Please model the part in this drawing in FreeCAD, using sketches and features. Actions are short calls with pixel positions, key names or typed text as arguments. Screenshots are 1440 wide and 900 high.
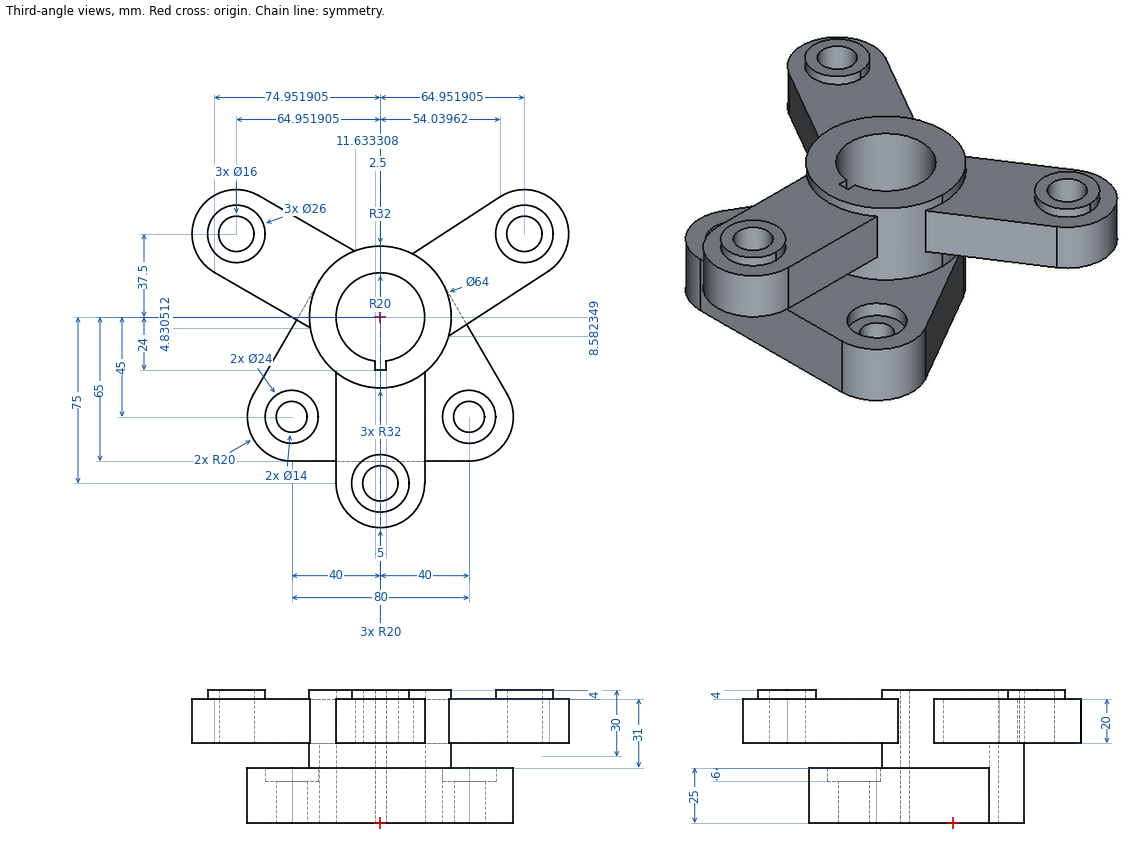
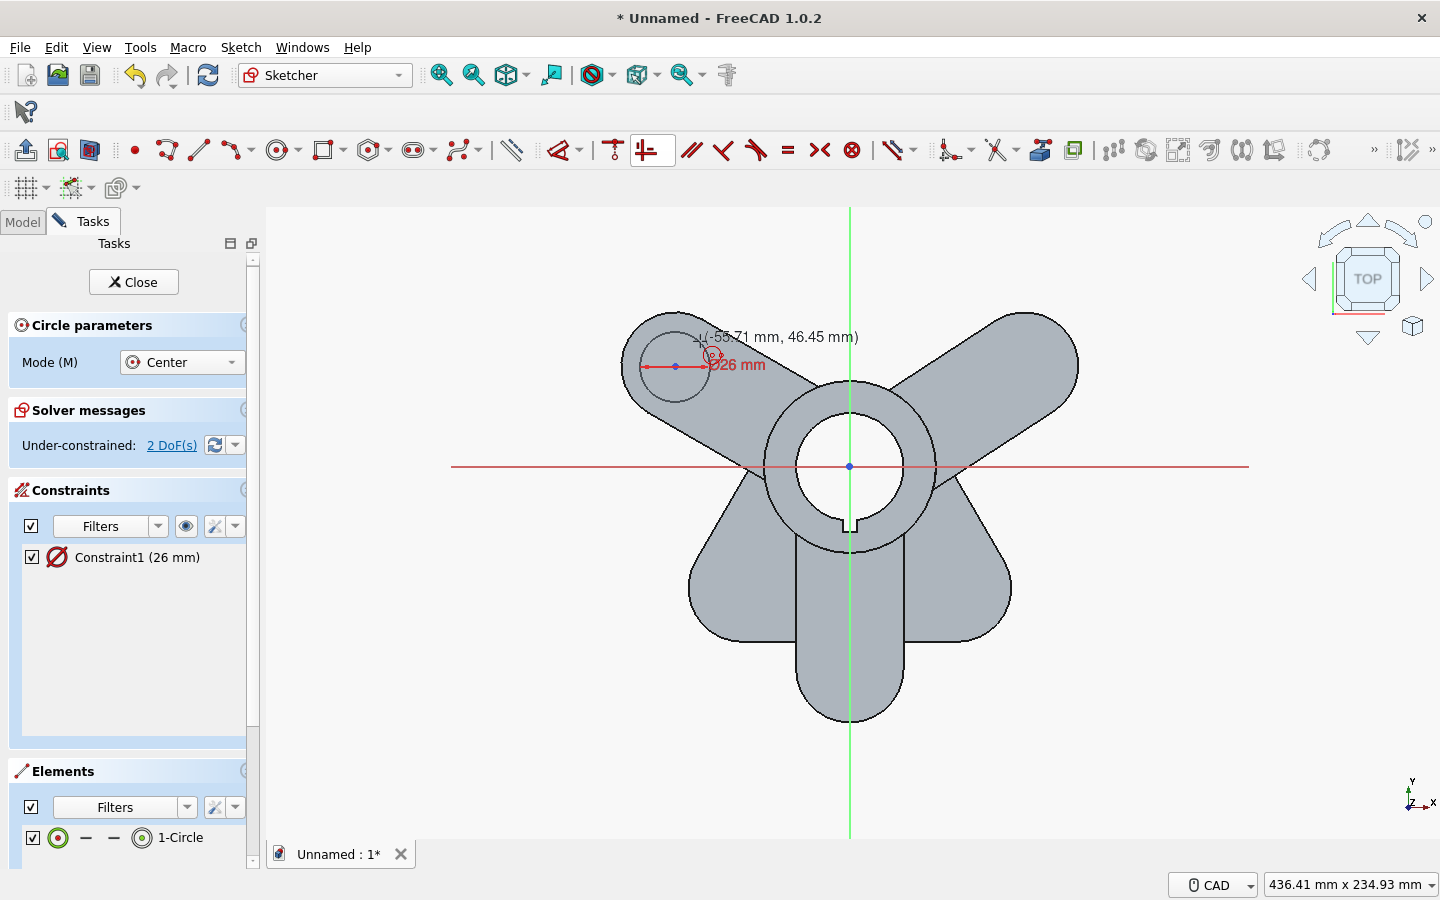
click(1025, 366)
move(1049, 341)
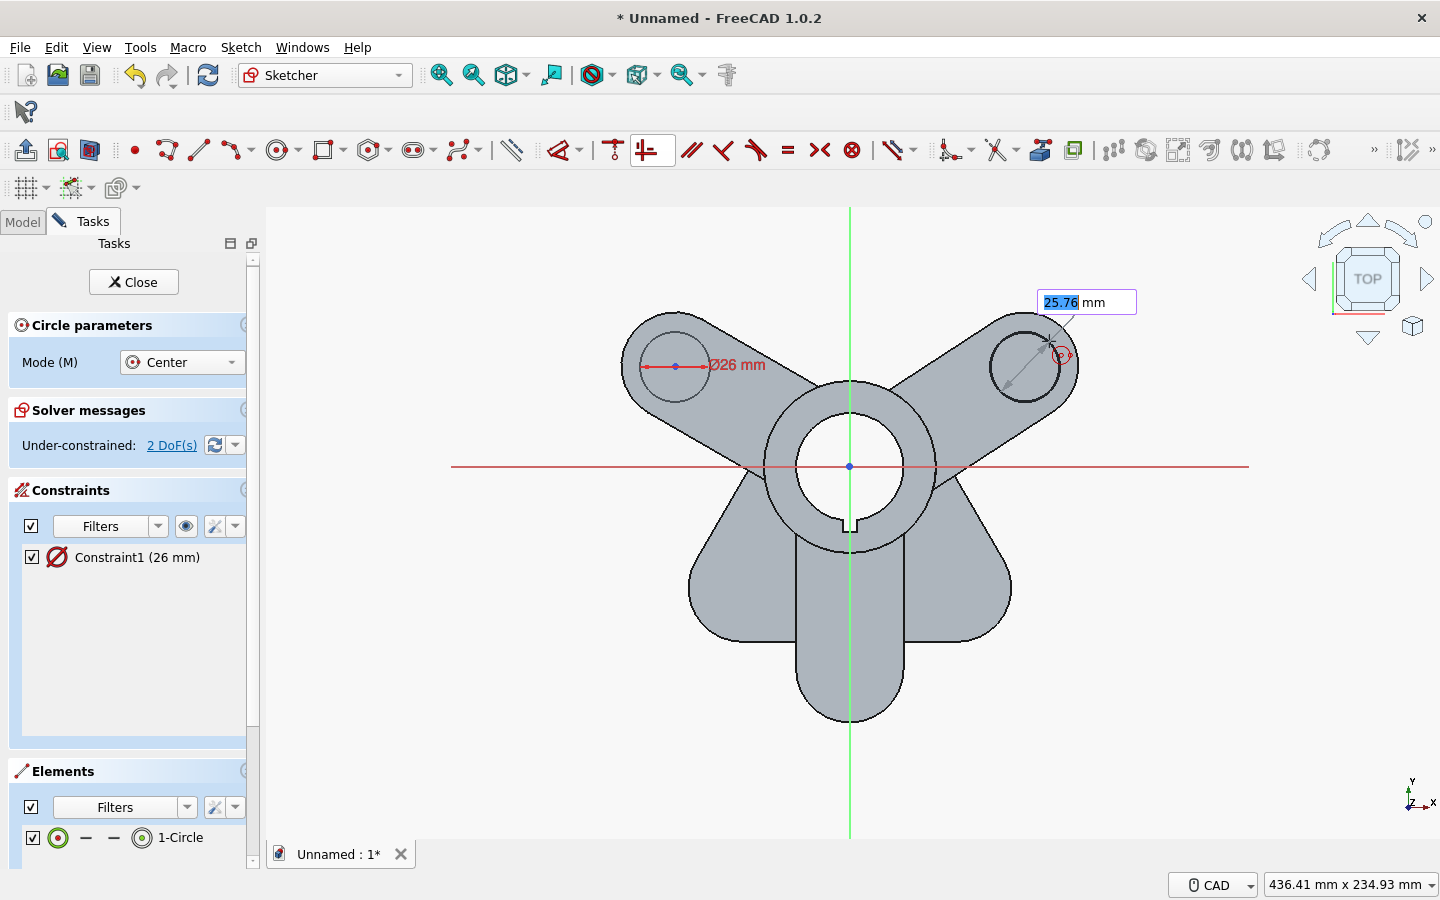
text(26)
key(Return)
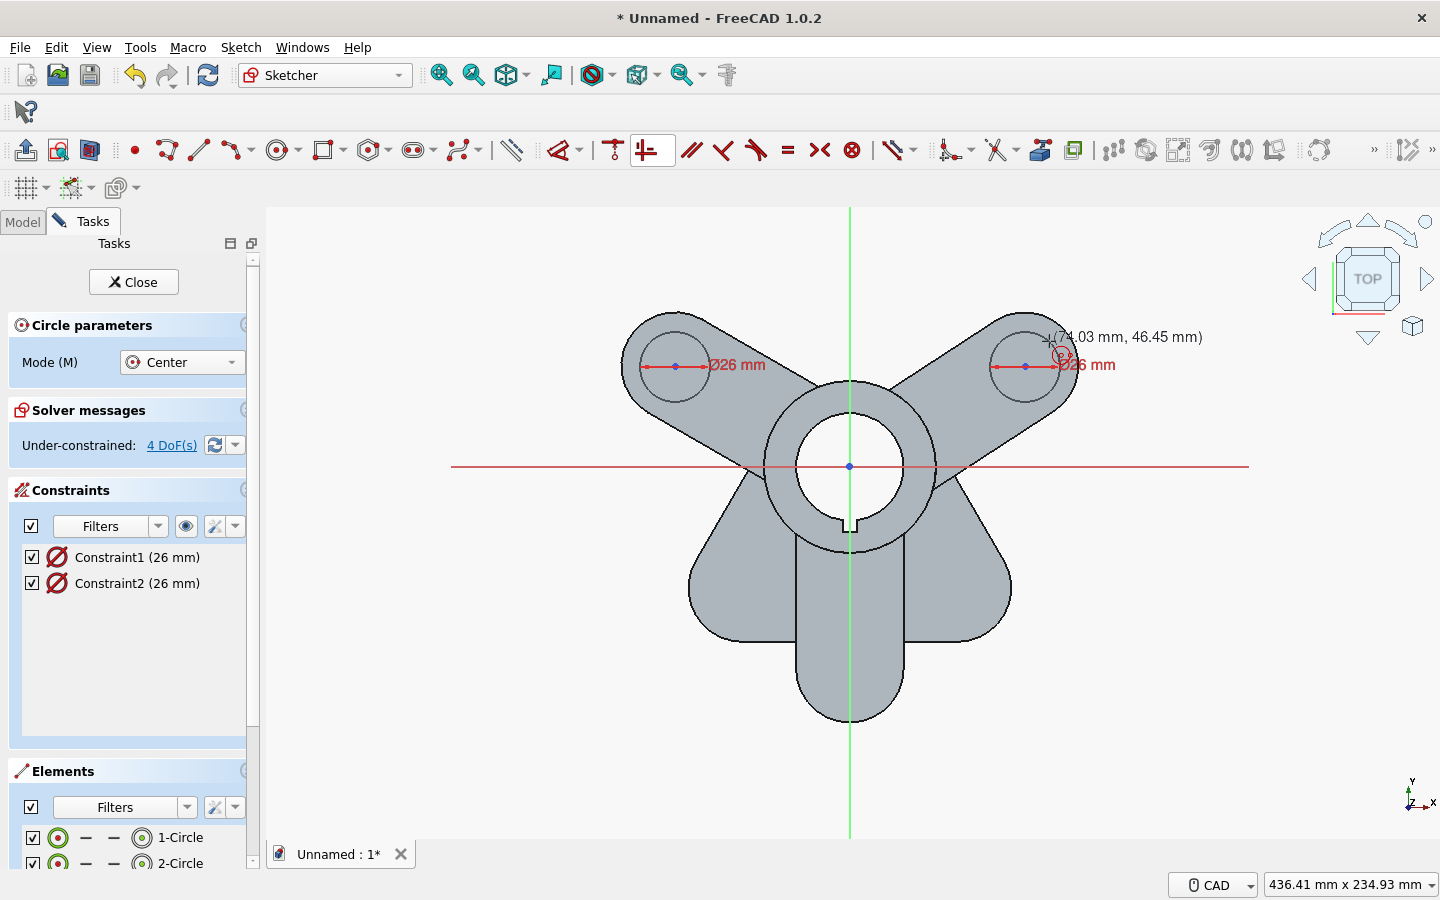
click(850, 669)
move(875, 644)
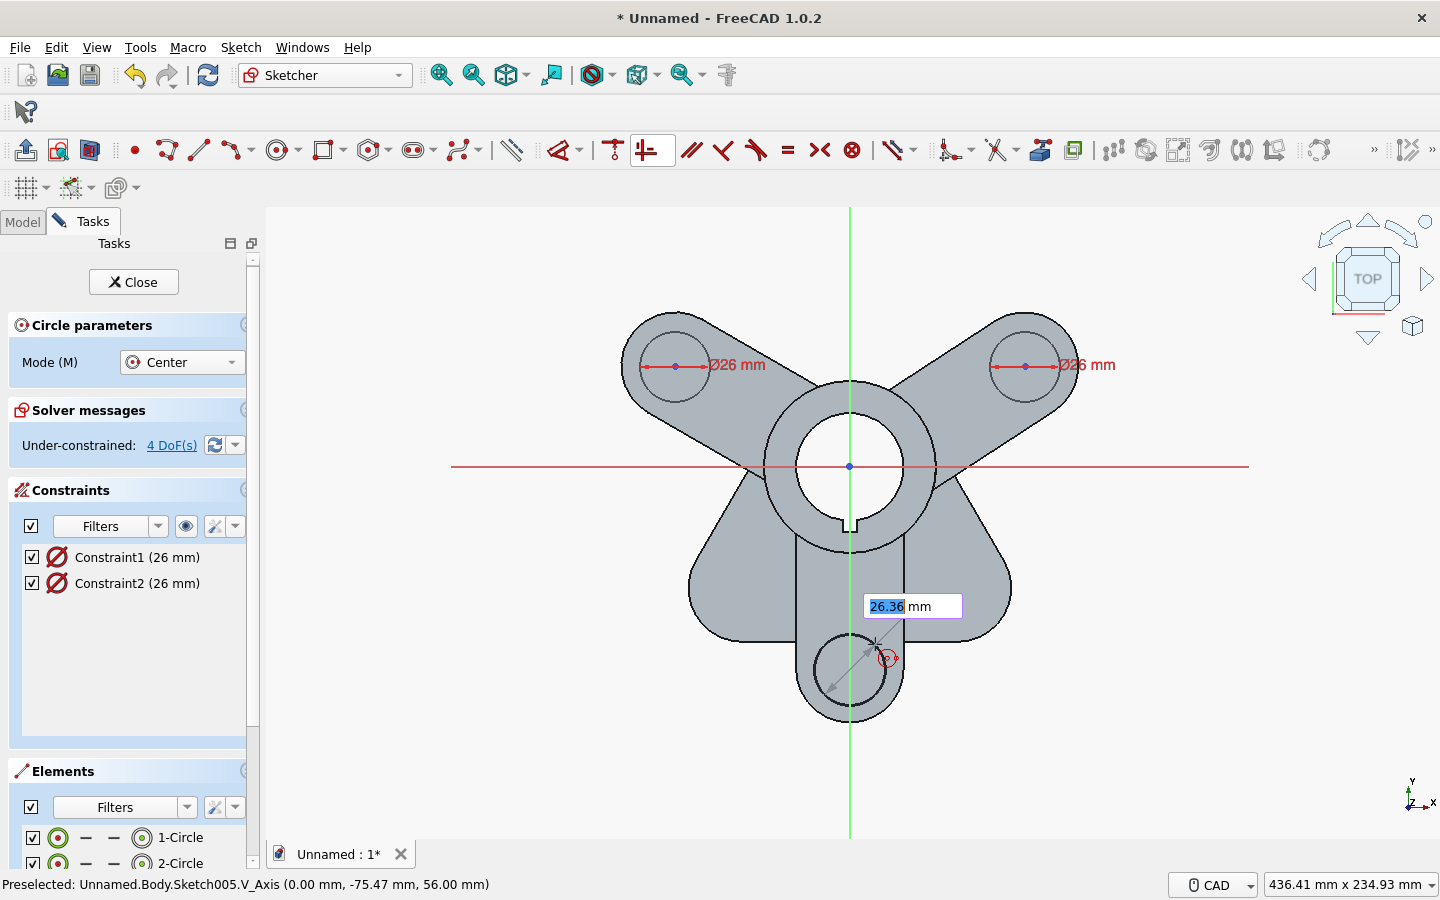
text(26)
key(Return)
key(Escape)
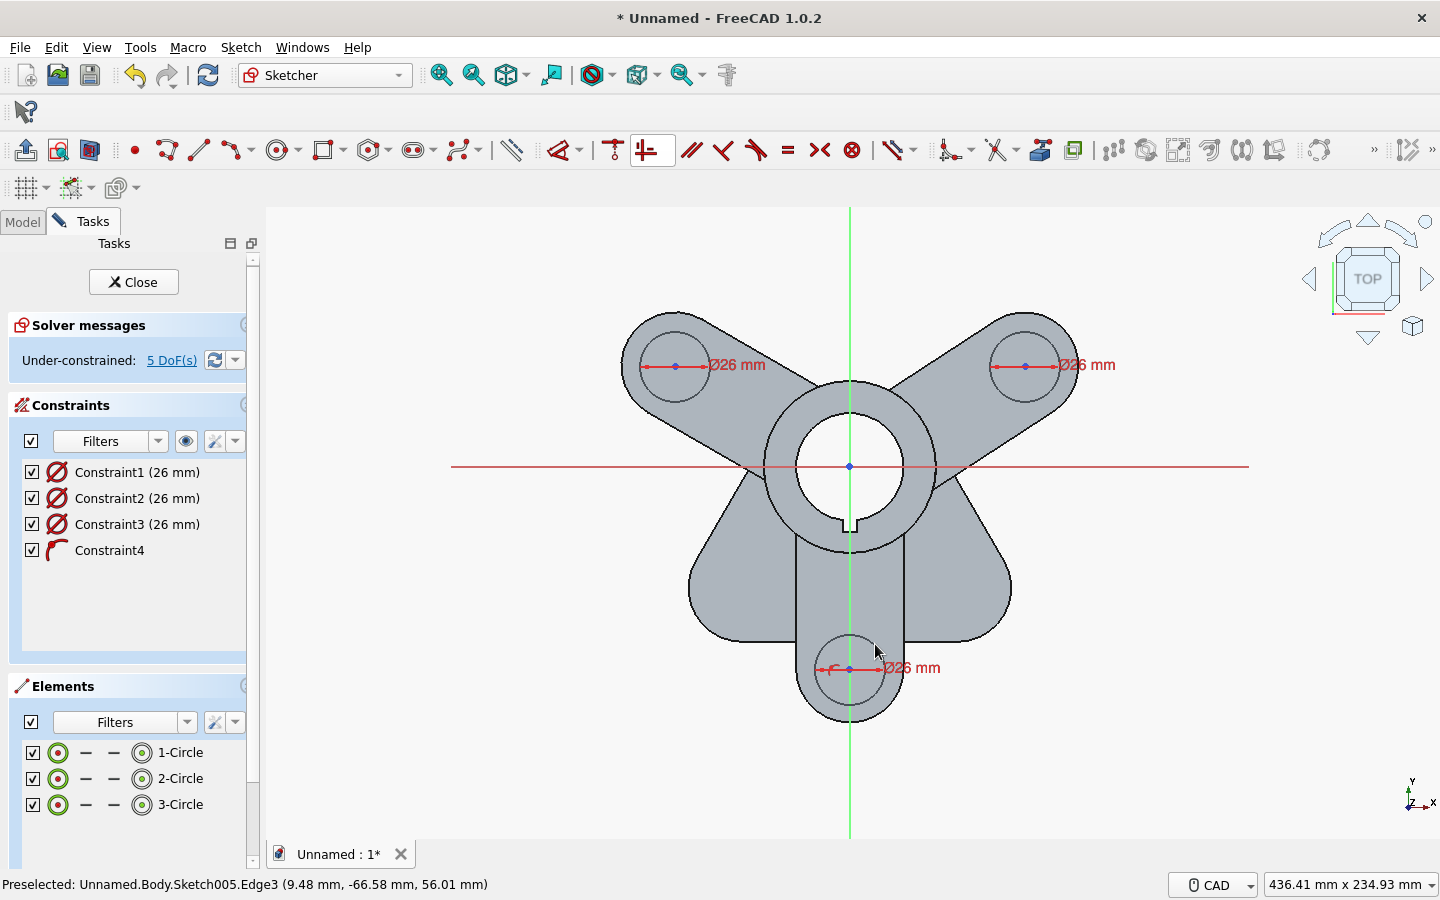
click(675, 367)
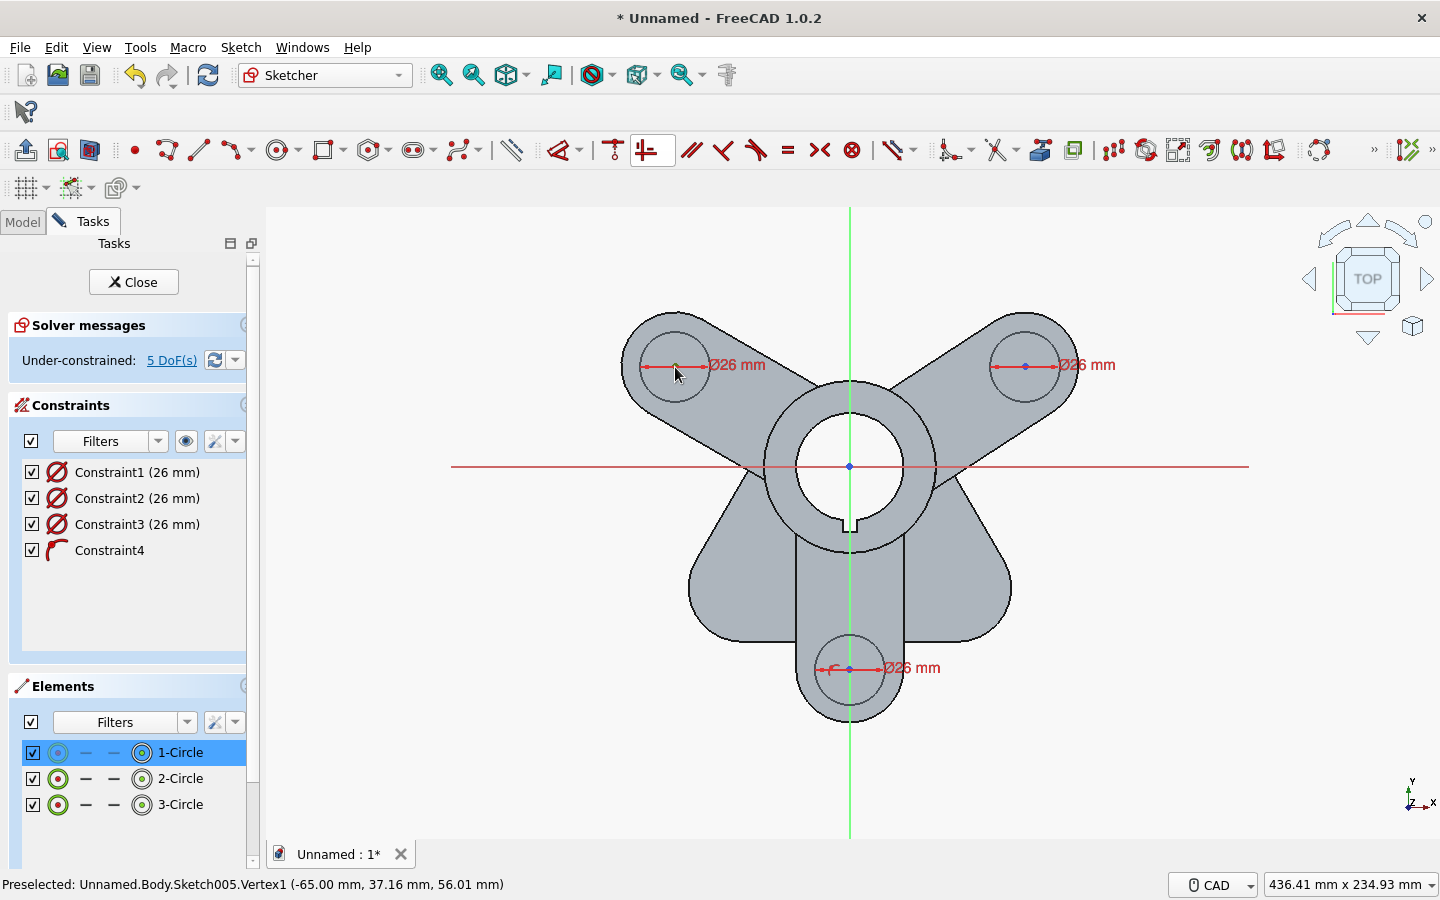
click(1025, 367)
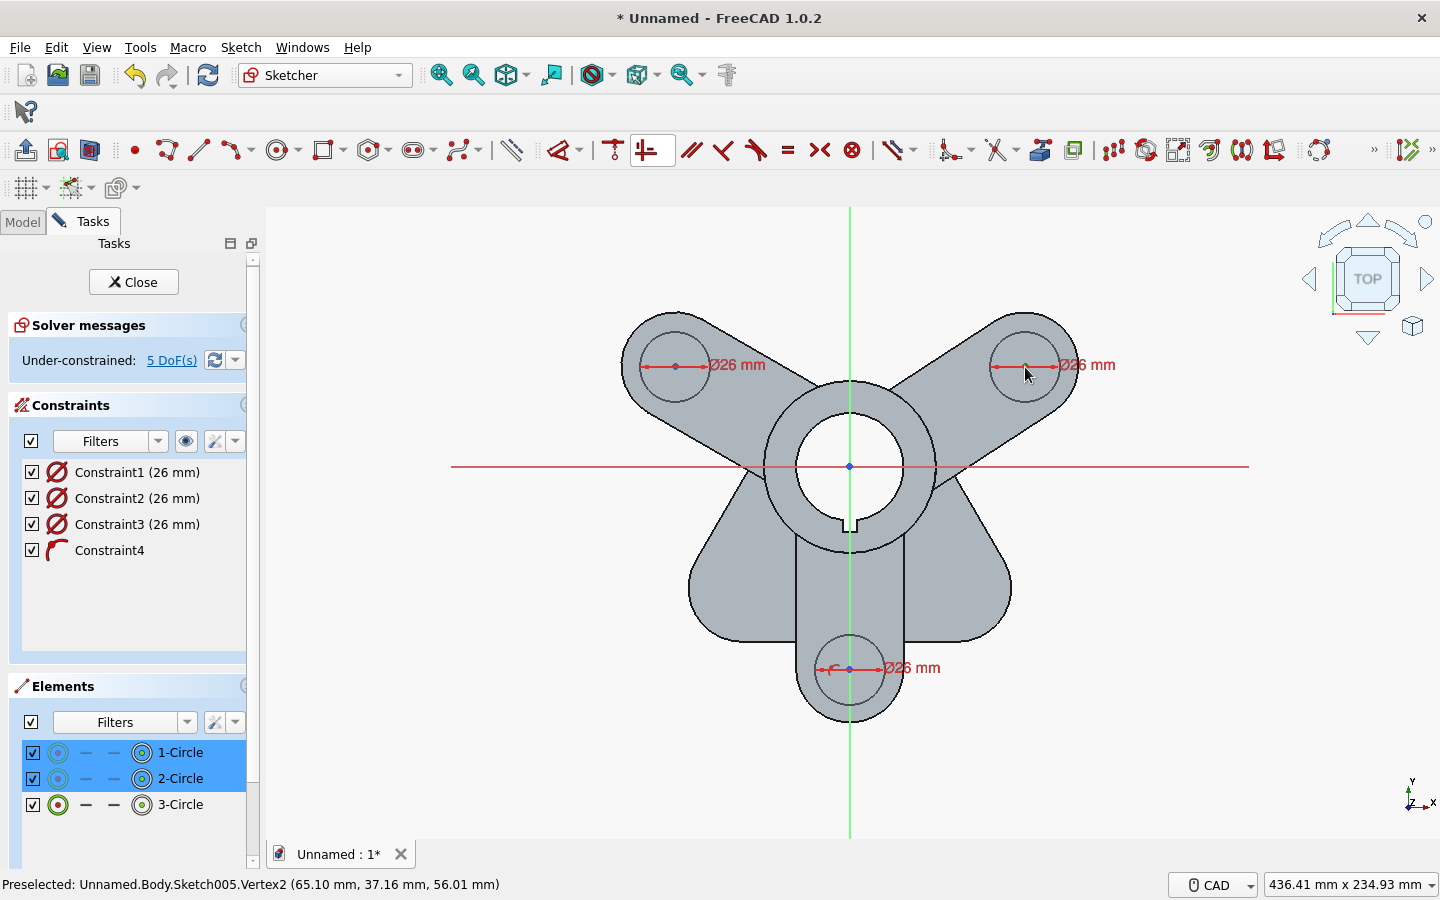
click(670, 150)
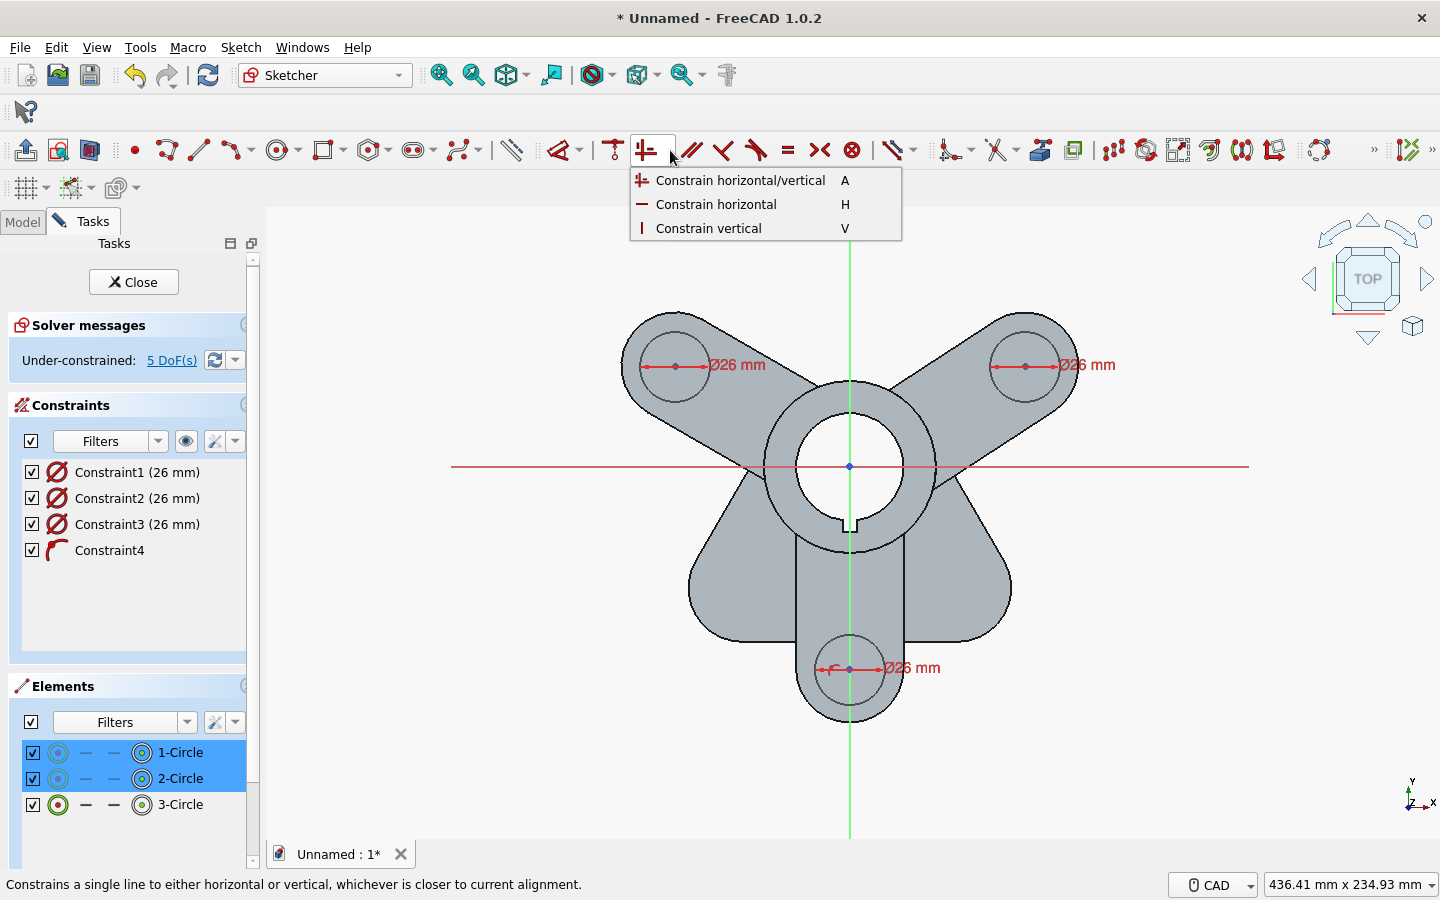
click(766, 204)